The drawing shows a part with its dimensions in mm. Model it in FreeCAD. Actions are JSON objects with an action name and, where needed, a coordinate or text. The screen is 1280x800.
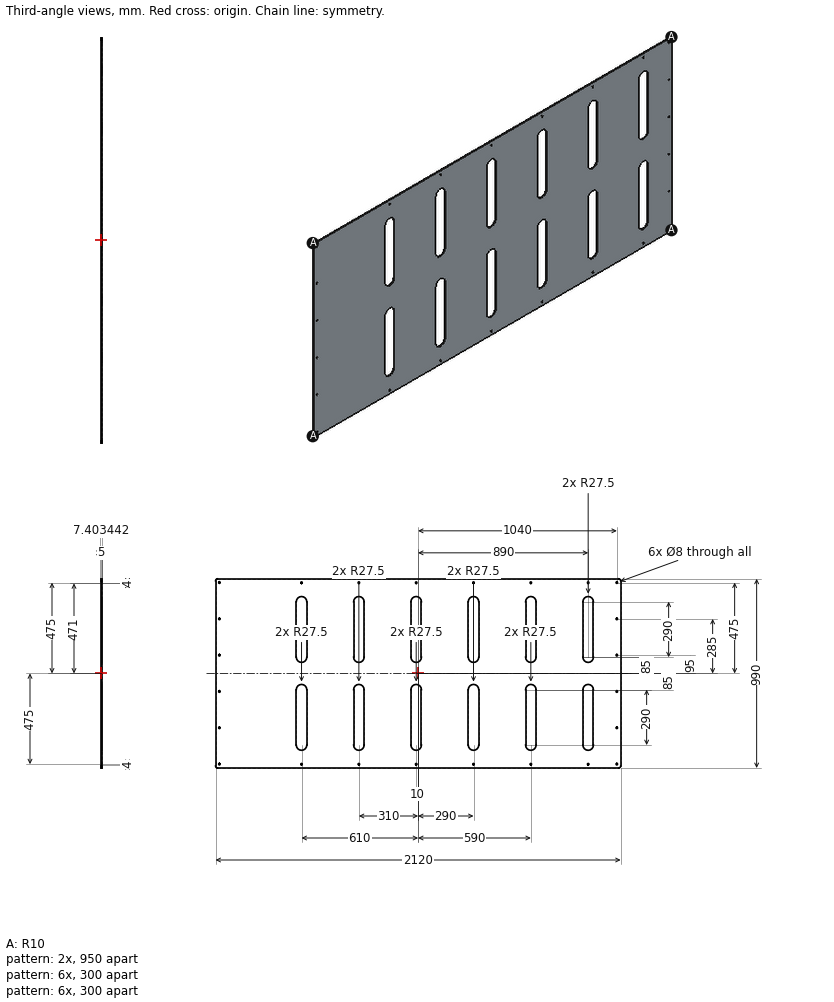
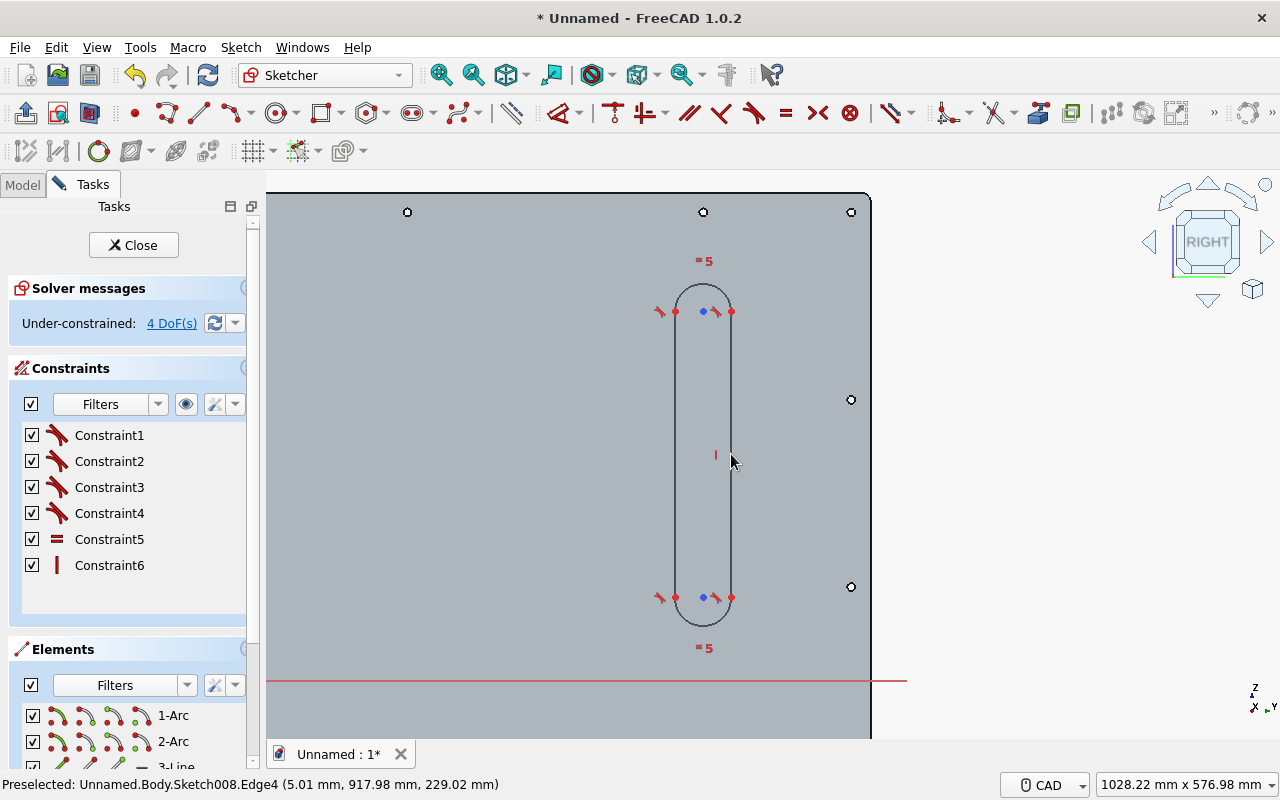
{"action": "left_click", "coordinate": [558, 114]}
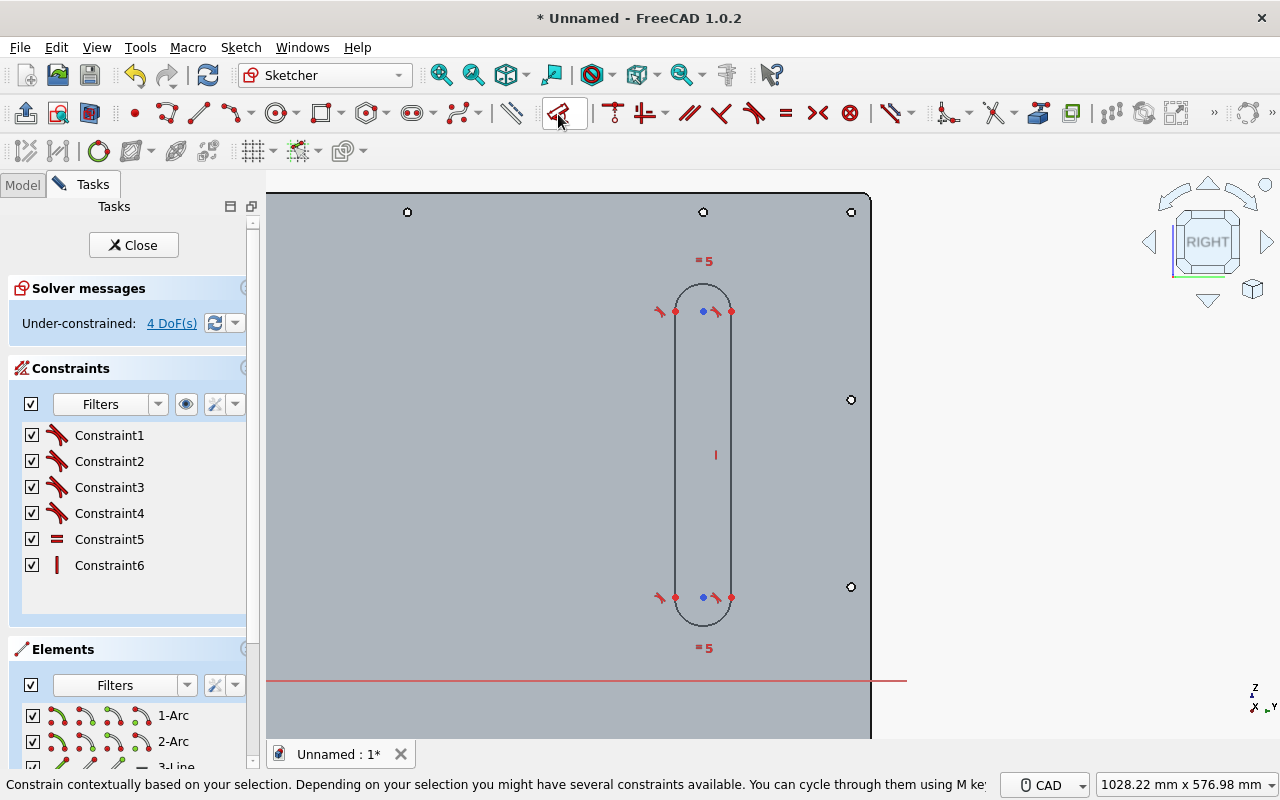
{"action": "scroll", "coordinate": [687, 621], "scroll_direction": "up", "scroll_amount": 2}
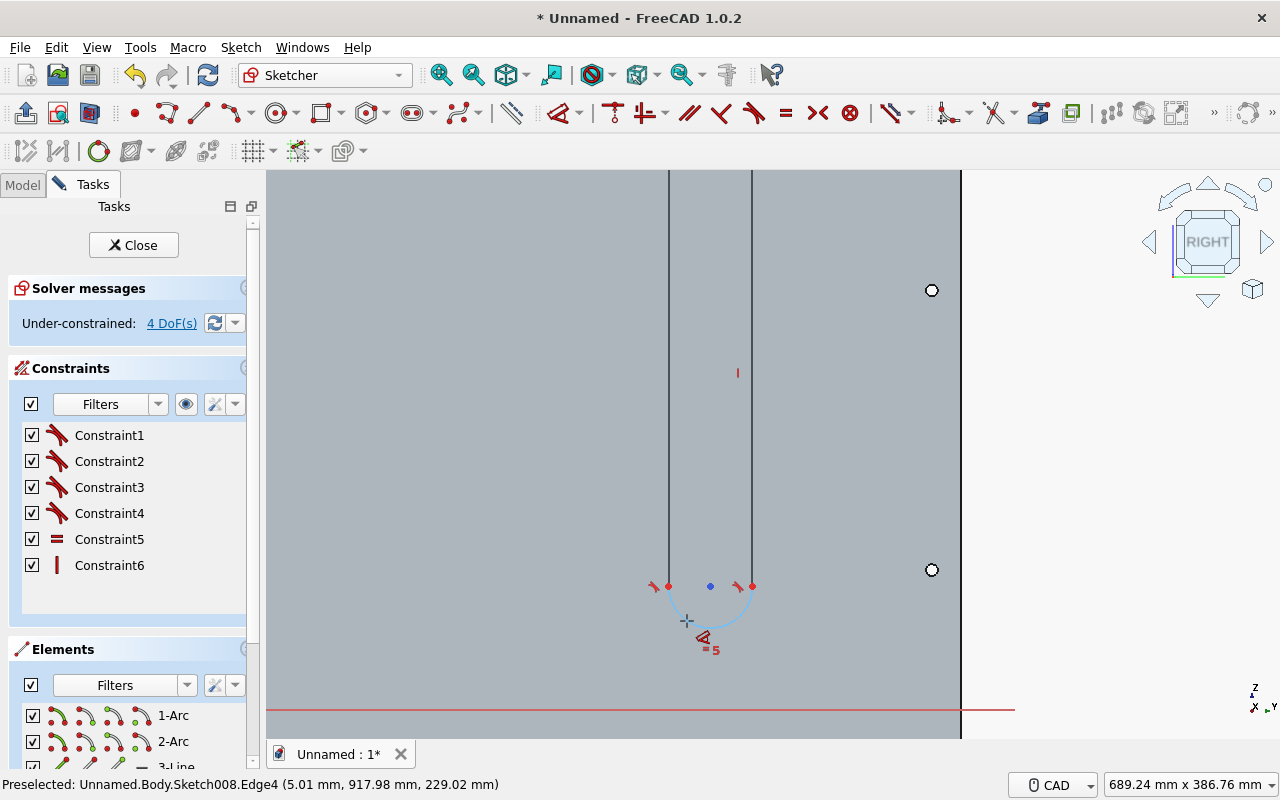
{"action": "left_click", "coordinate": [686, 620]}
{"action": "left_click", "coordinate": [667, 646]}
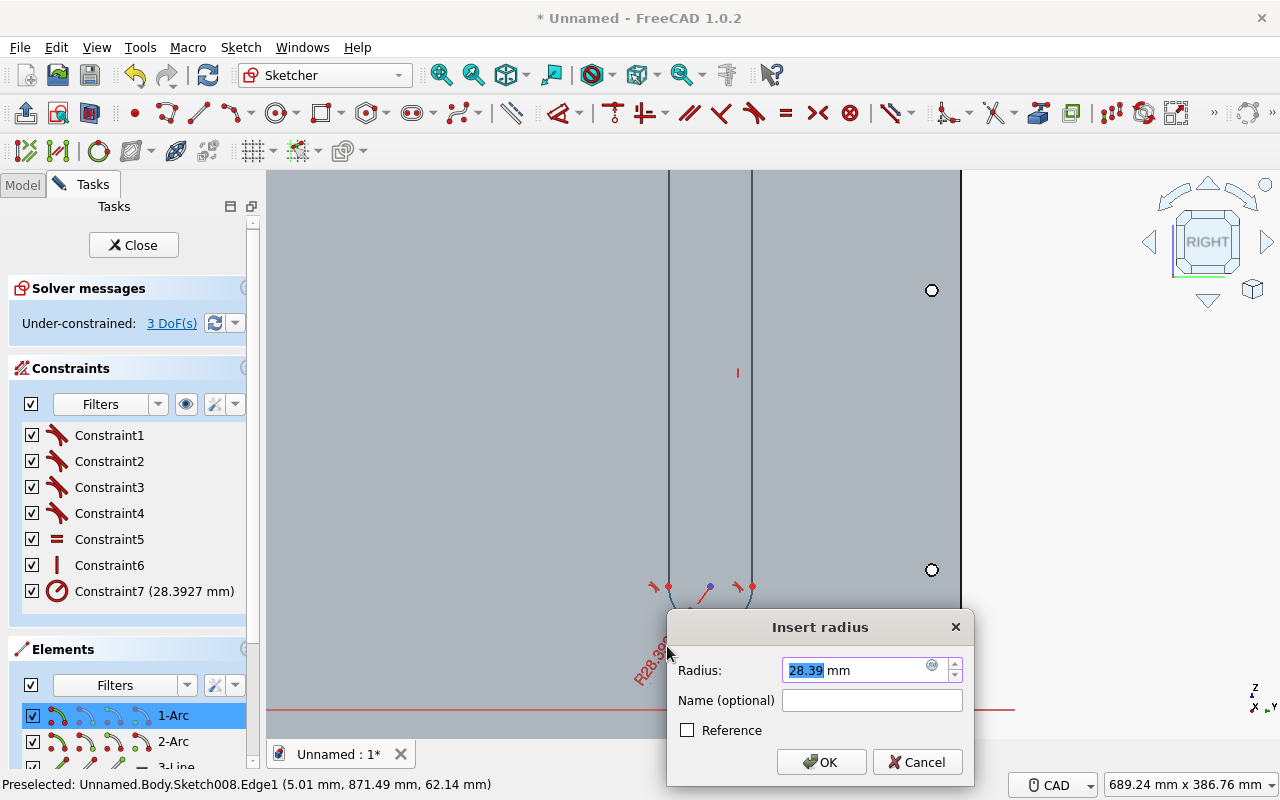
{"action": "type", "text": "27.5"}
{"action": "key", "text": "Return"}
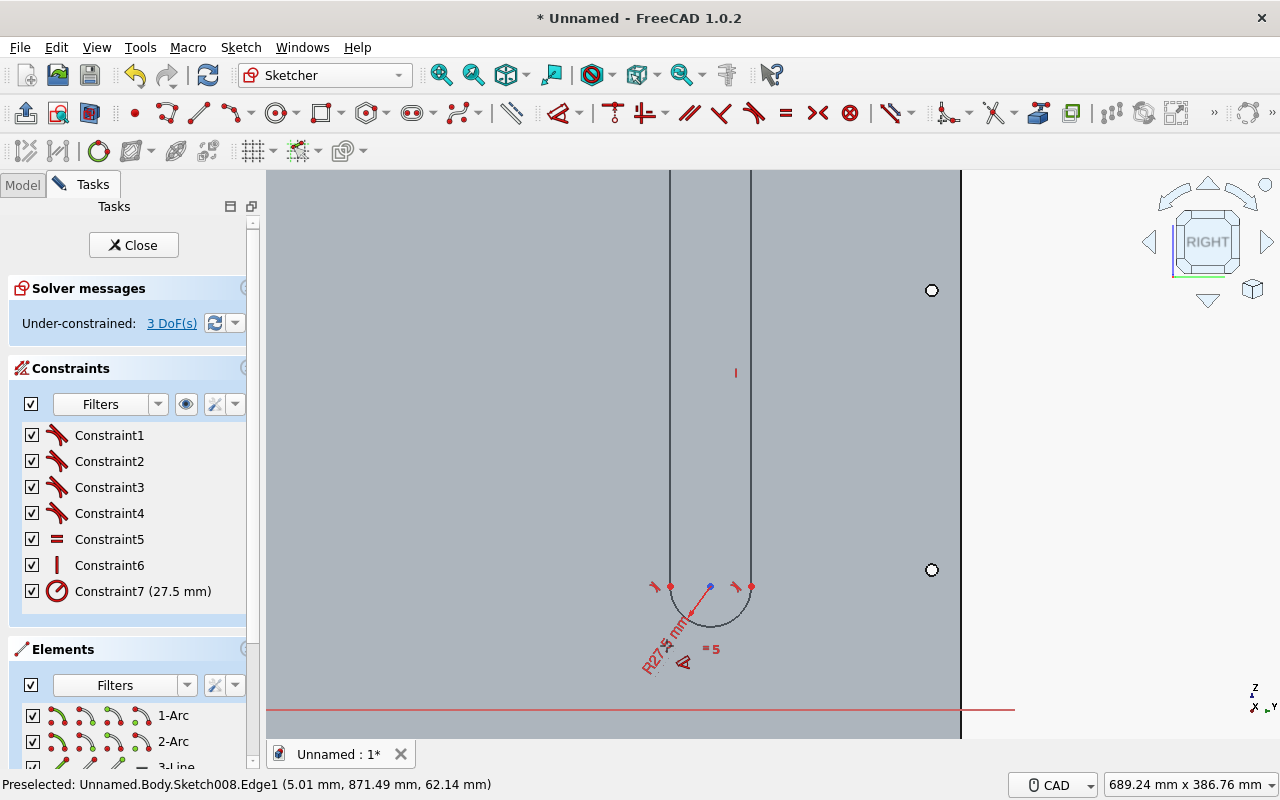
{"action": "left_click", "coordinate": [670, 458]}
{"action": "left_click", "coordinate": [636, 392]}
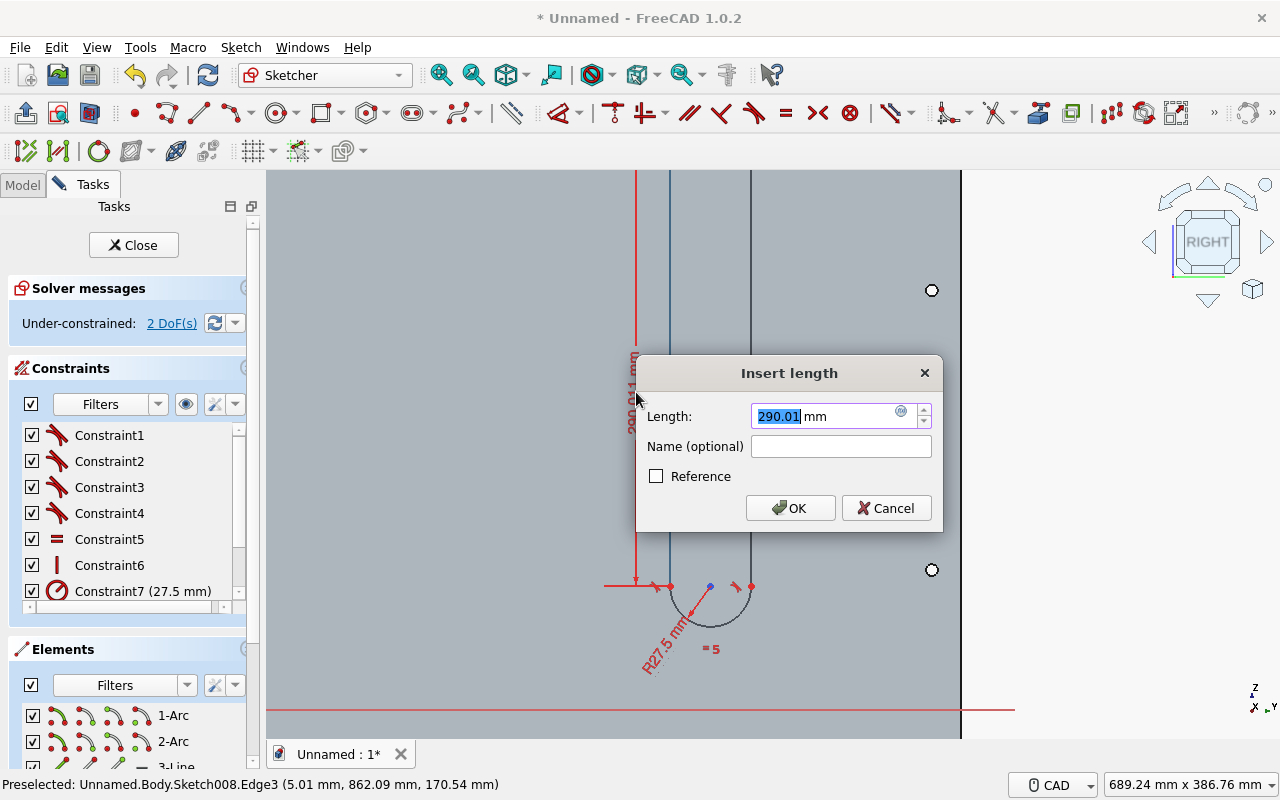
{"action": "type", "text": "290"}
{"action": "key", "text": "Return"}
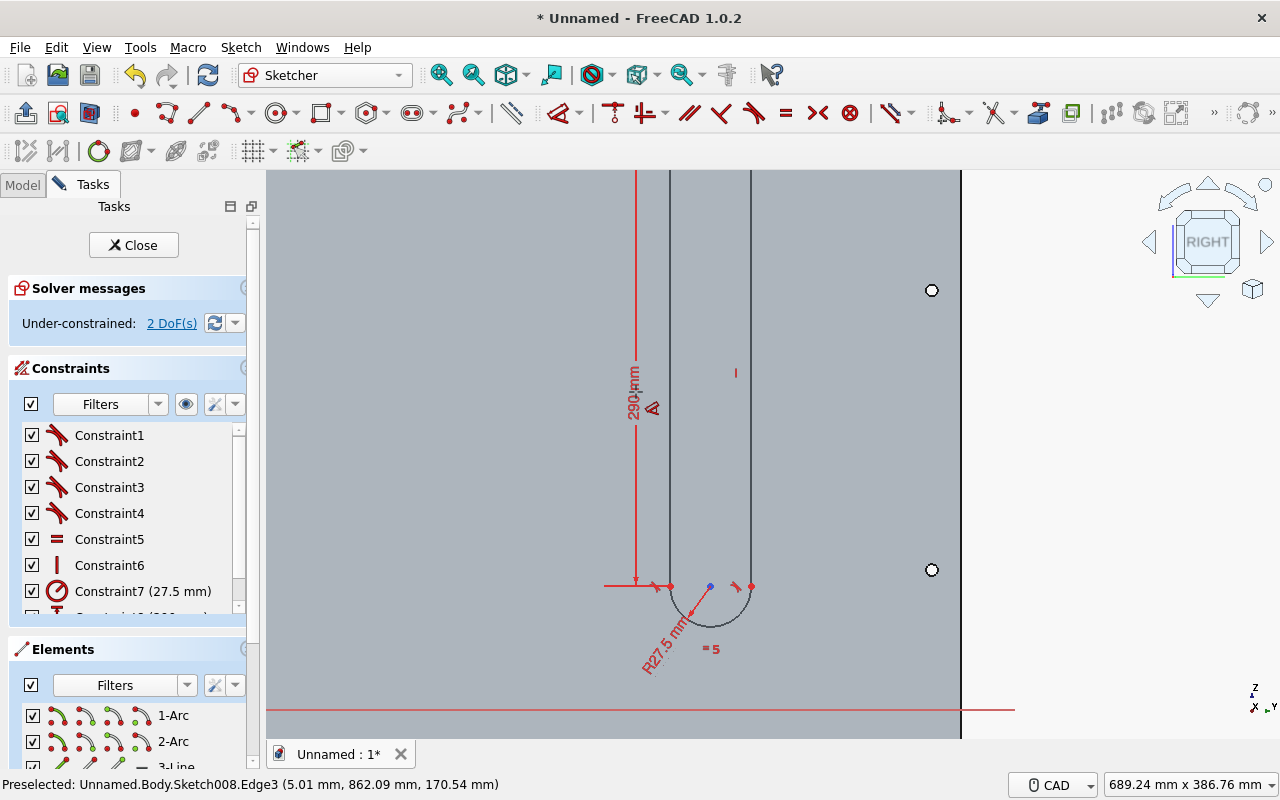
{"action": "left_click", "coordinate": [670, 586]}
{"action": "left_click", "coordinate": [704, 677]}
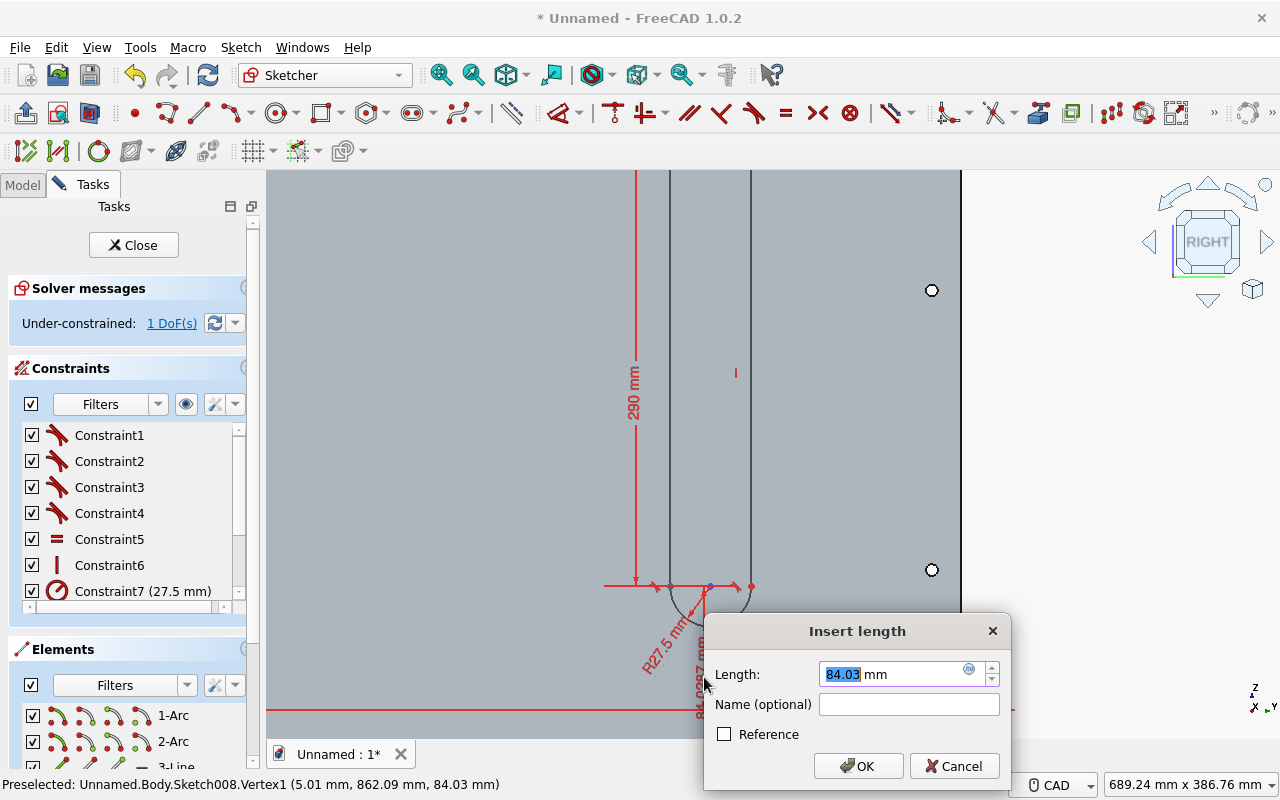
{"action": "type", "text": "85"}
{"action": "key", "text": "Return"}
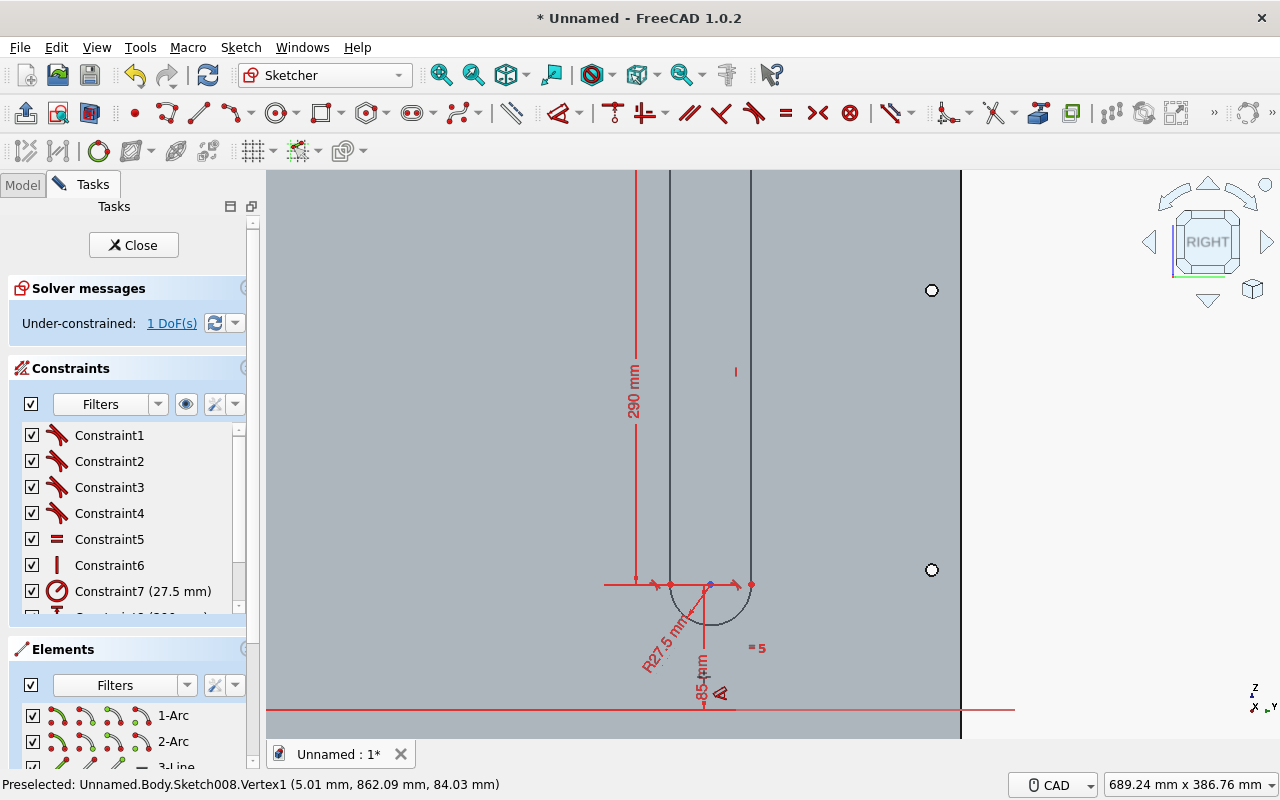
{"action": "left_click", "coordinate": [711, 585]}
{"action": "left_click", "coordinate": [502, 551]}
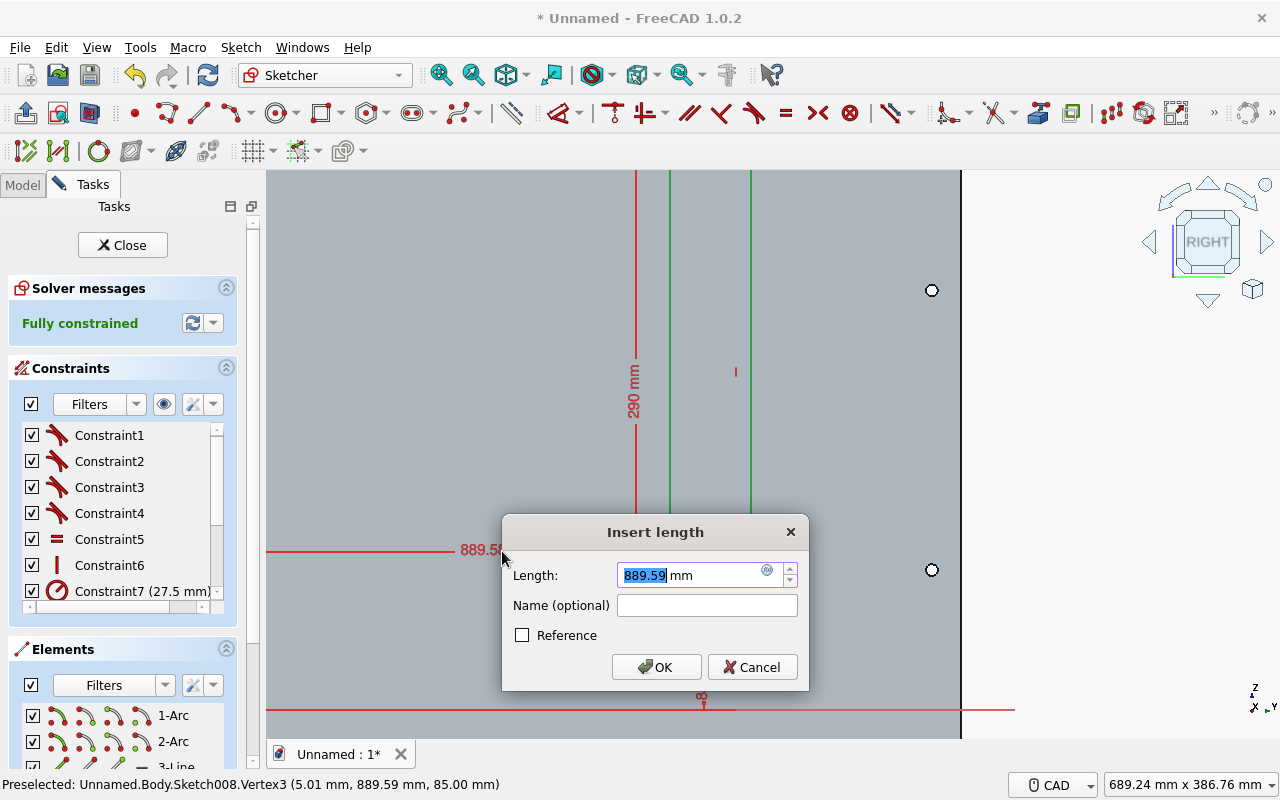
{"action": "type", "text": "890"}
{"action": "key", "text": "Return"}
{"action": "key", "text": "Escape"}